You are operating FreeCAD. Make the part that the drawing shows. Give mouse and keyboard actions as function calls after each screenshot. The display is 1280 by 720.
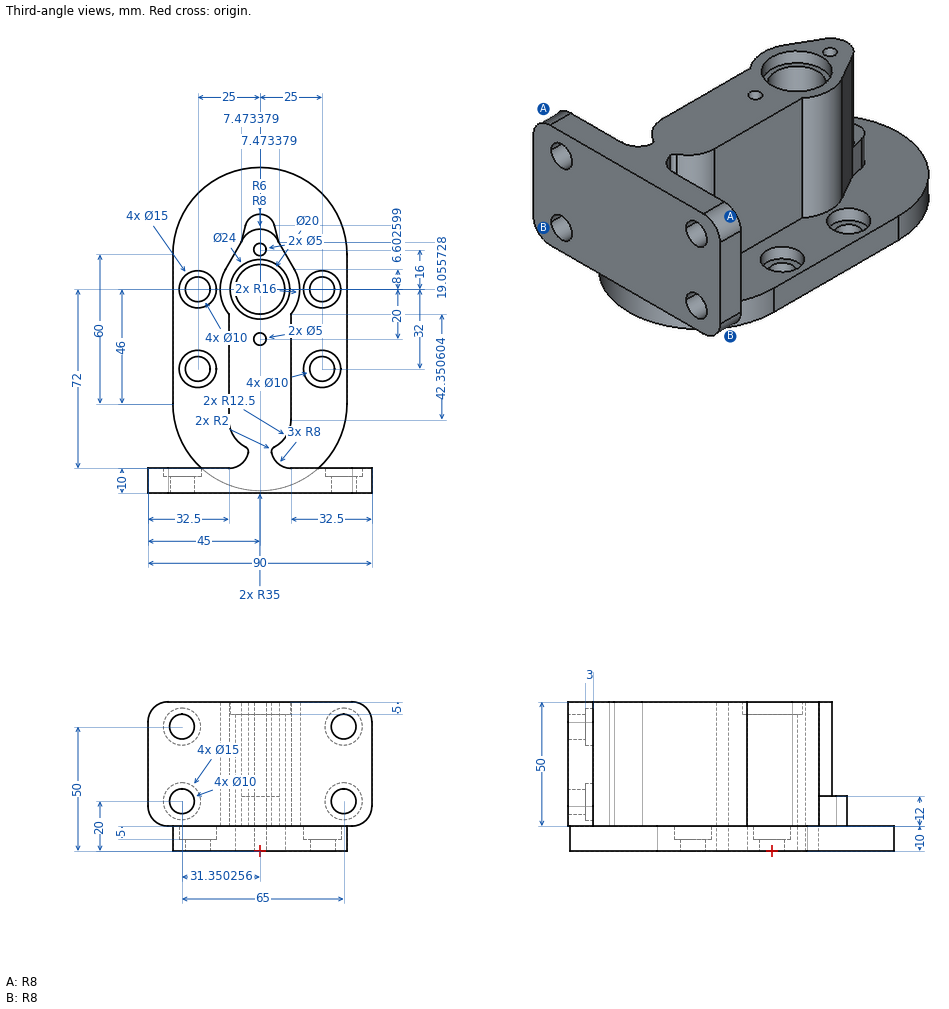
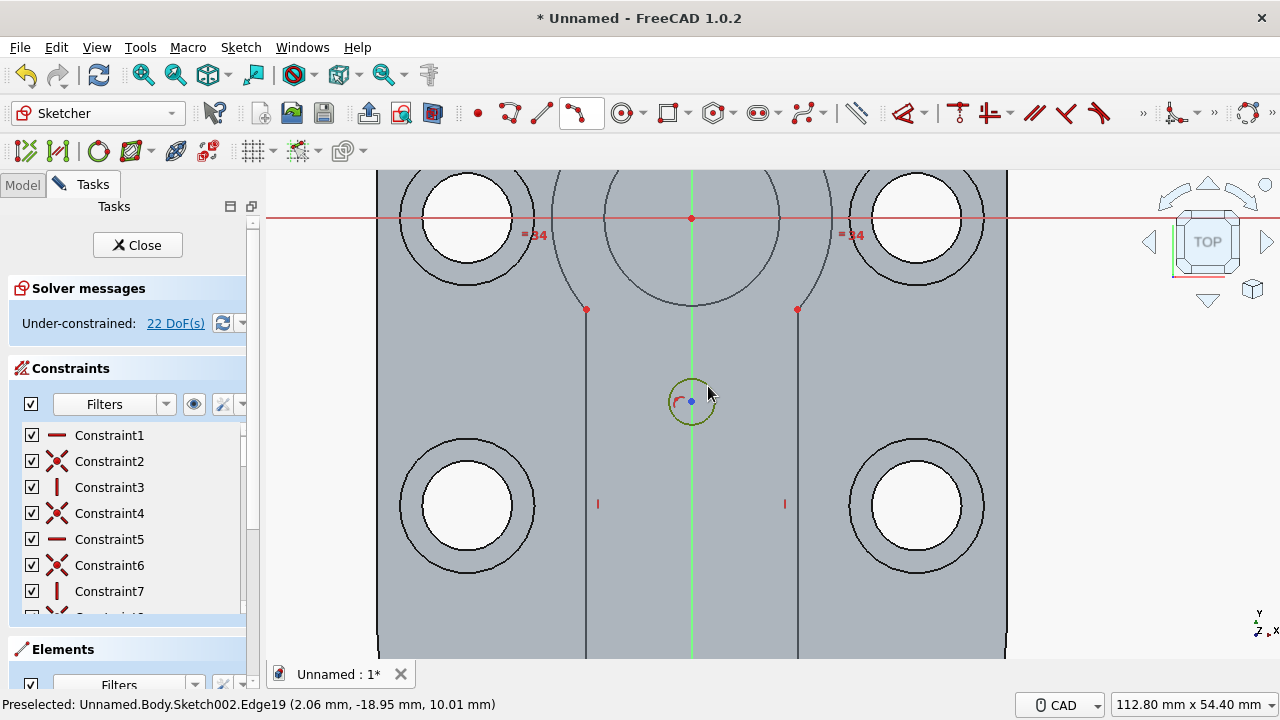
scroll(710, 387, down, 6)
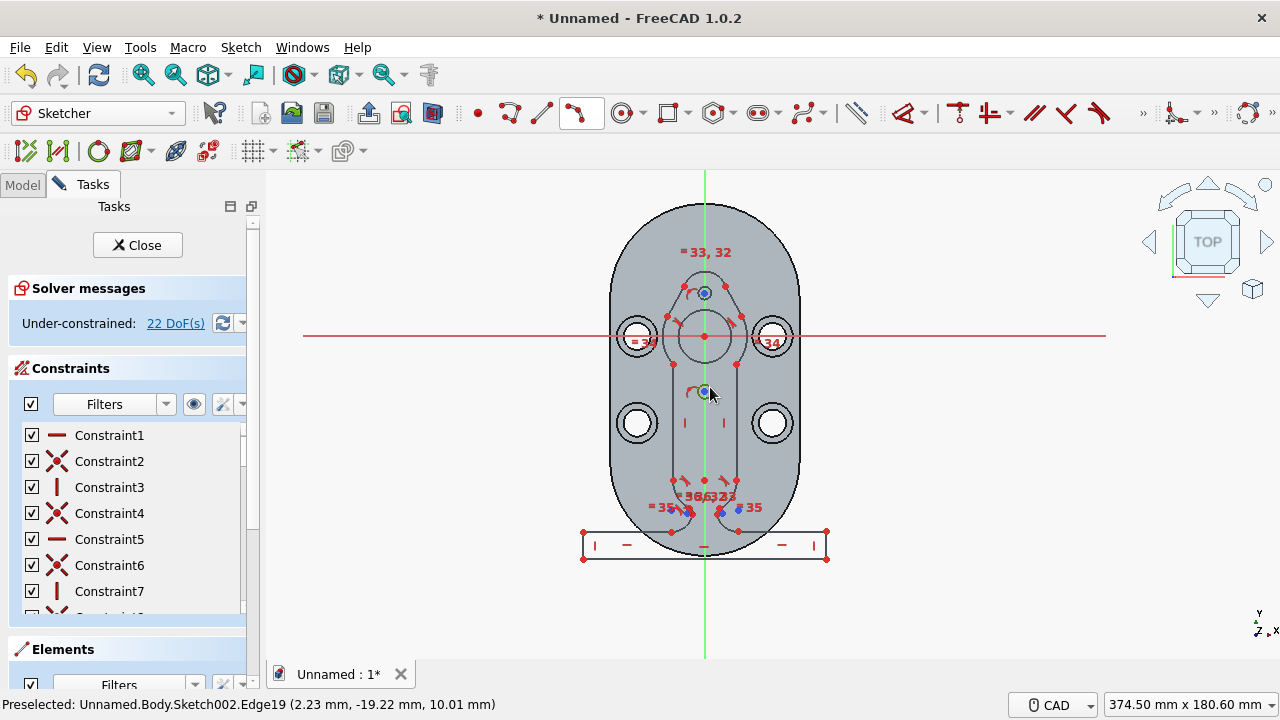
scroll(709, 289, up, 6)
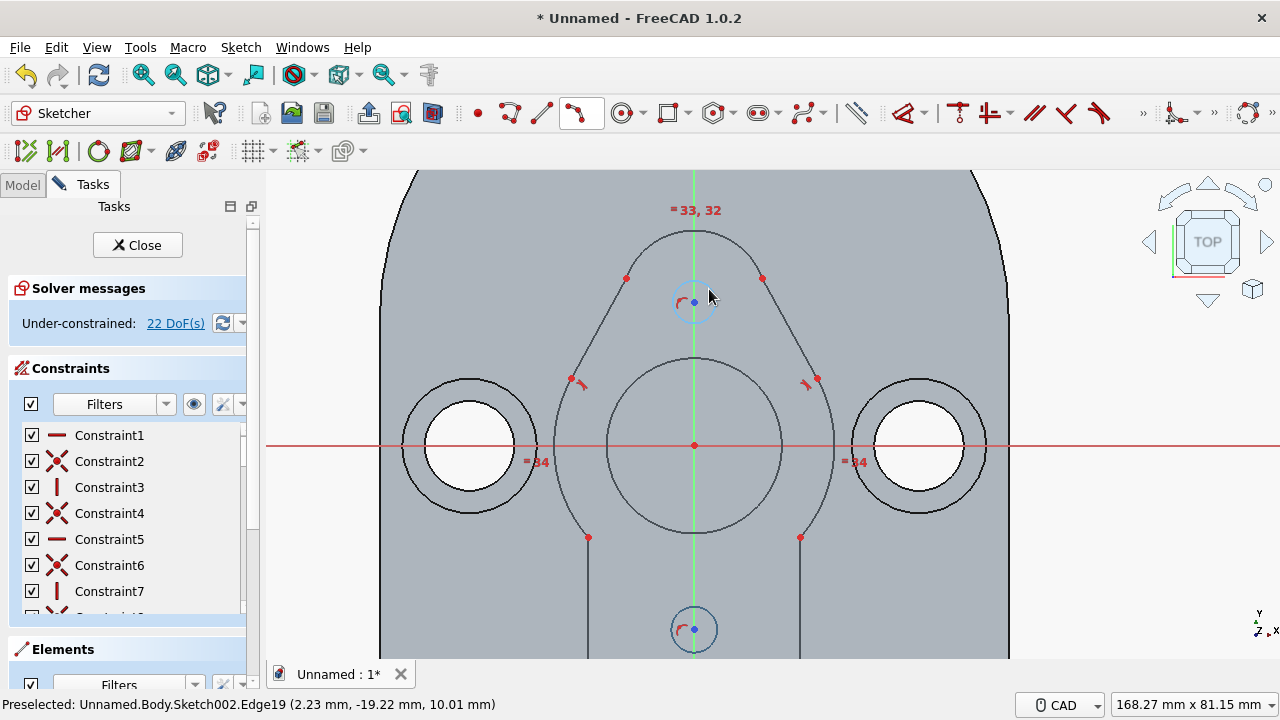
click(709, 287)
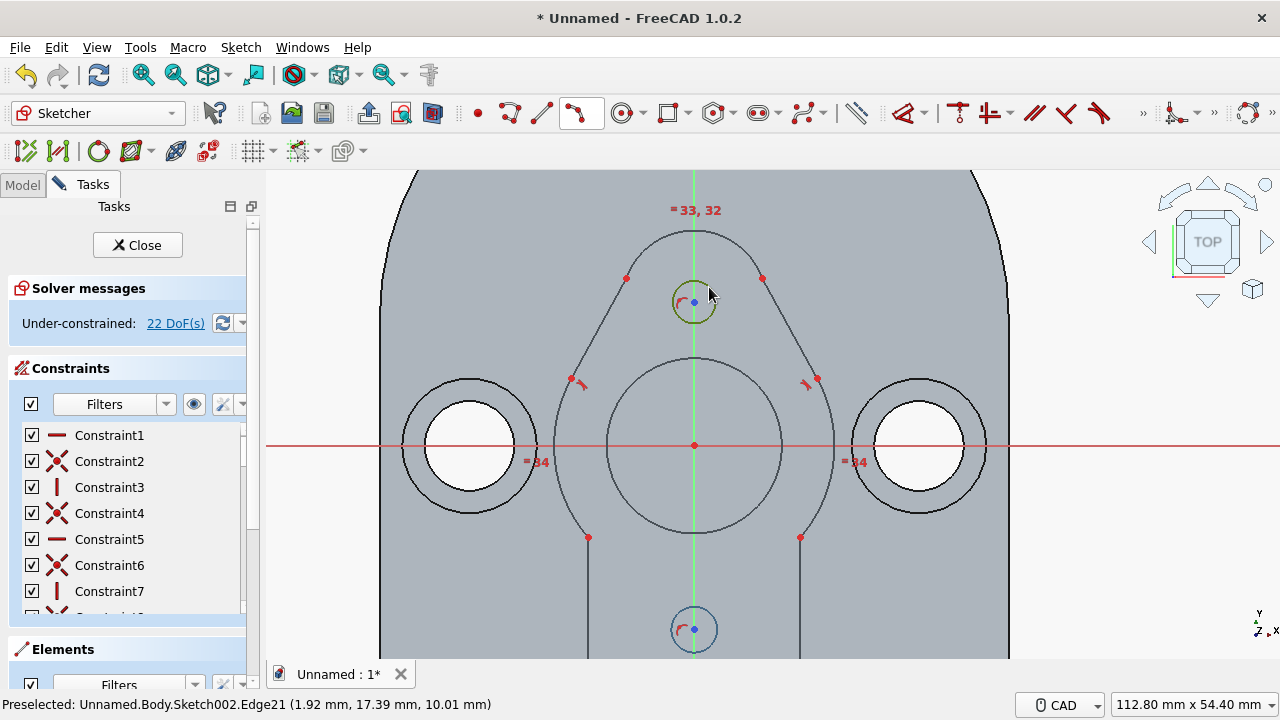
key(e)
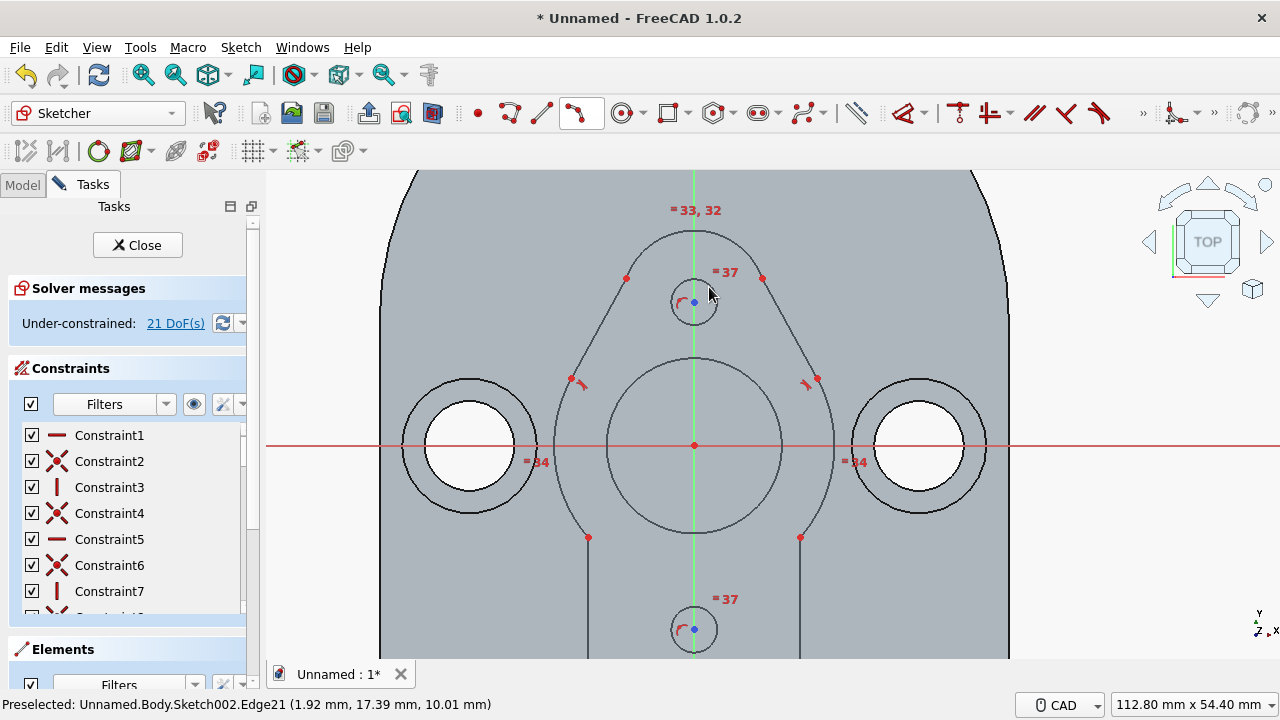
scroll(709, 289, down, 6)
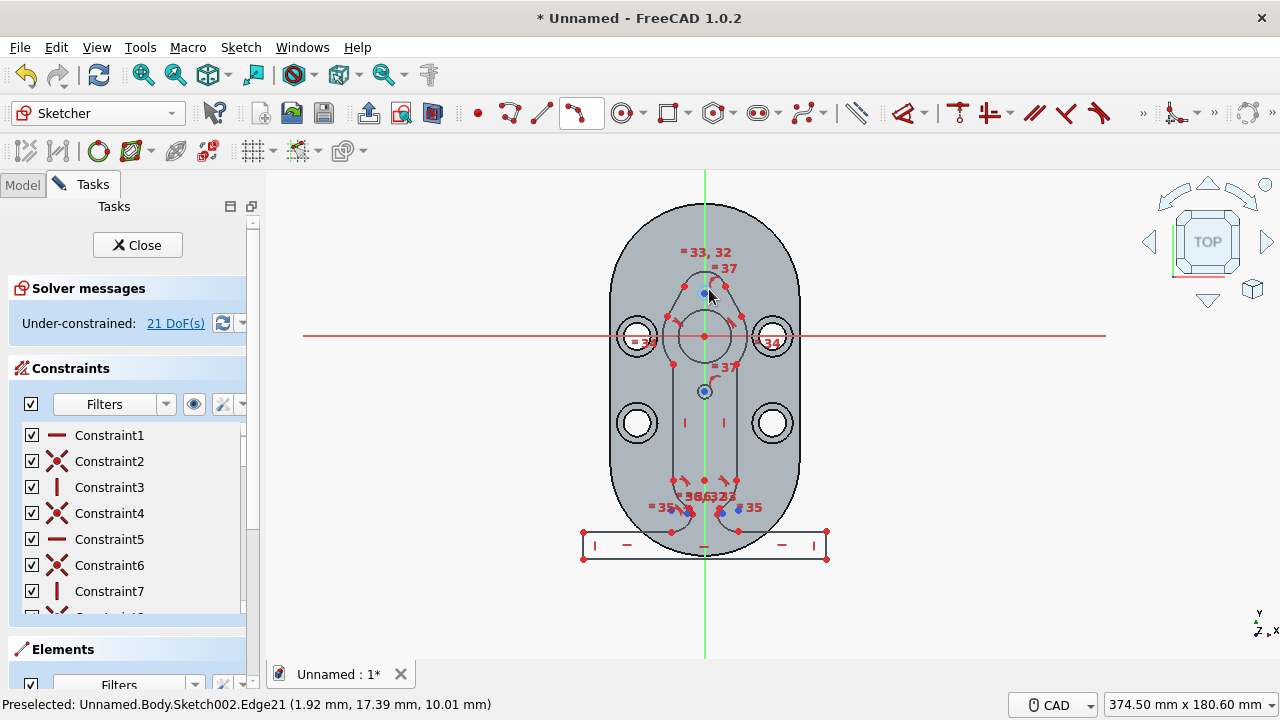
click(705, 481)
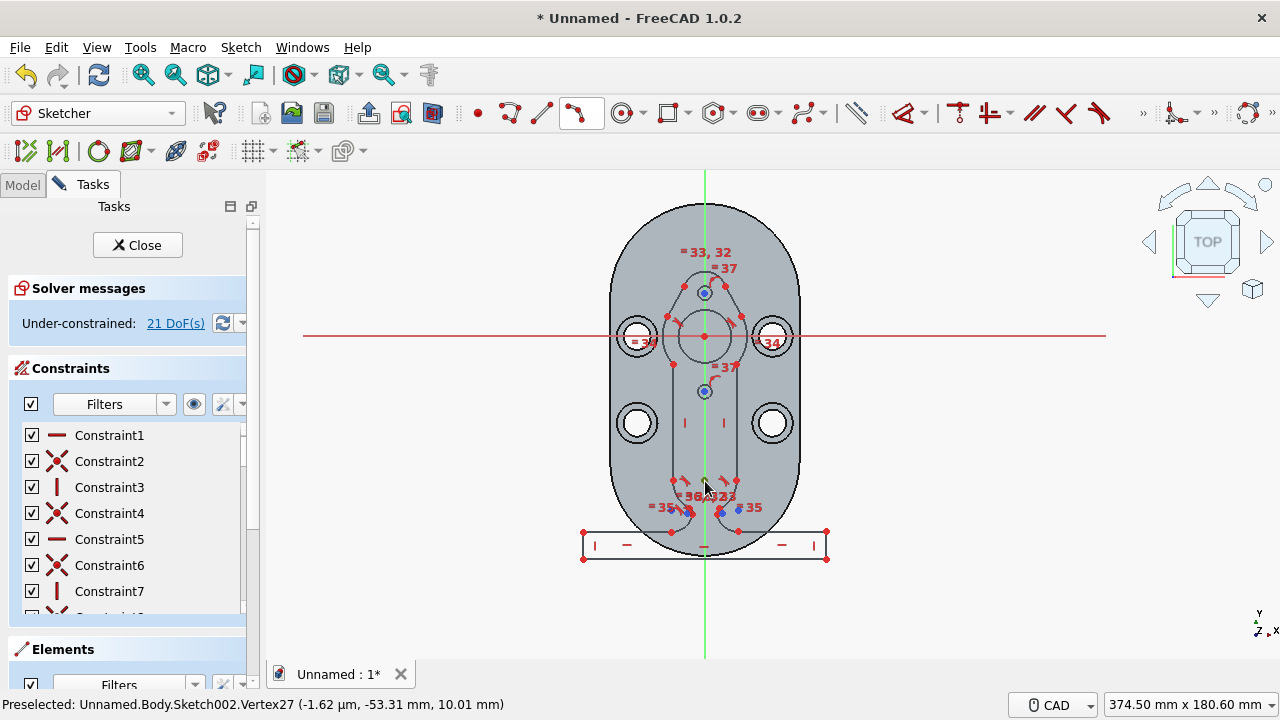
click(705, 600)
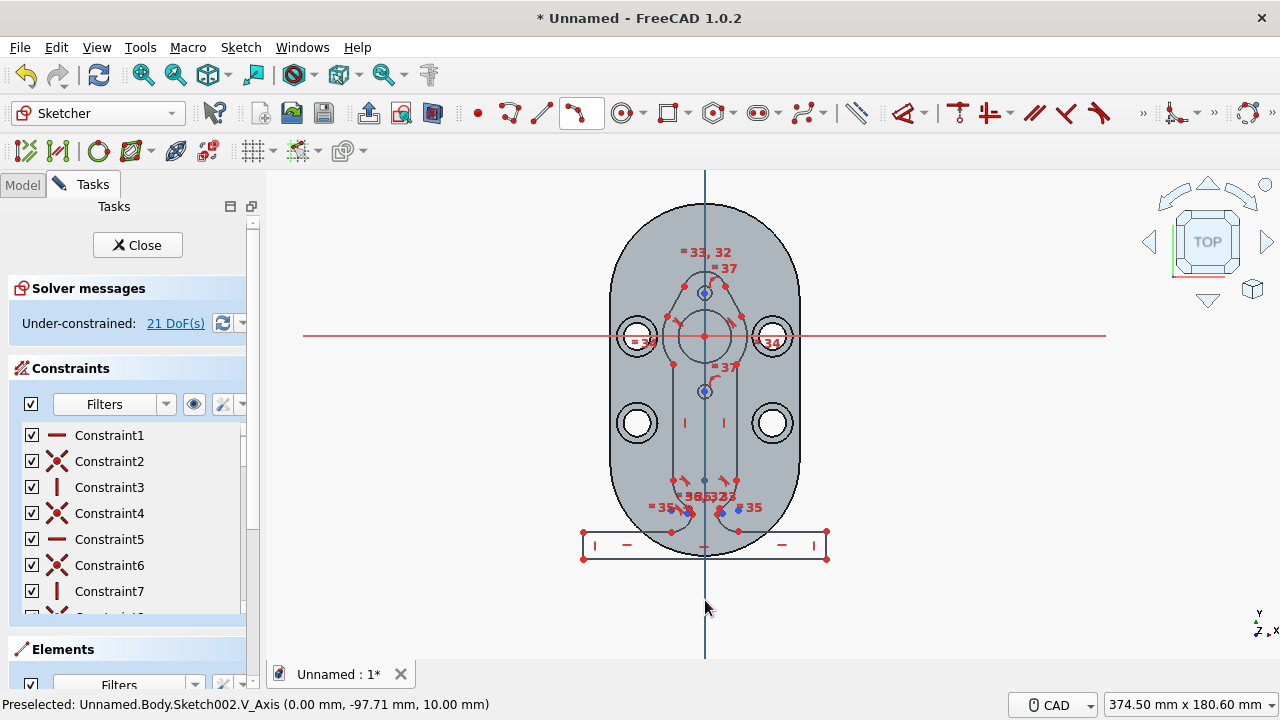
click(958, 114)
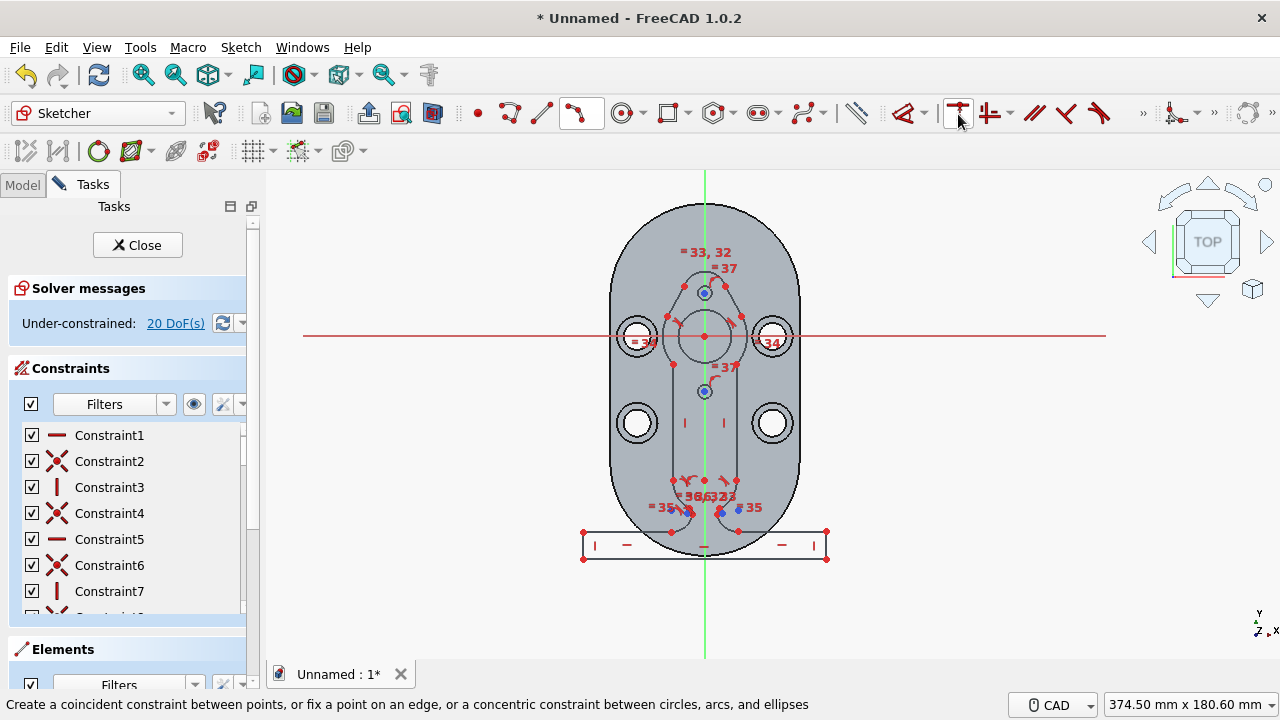
scroll(705, 293, up, 14)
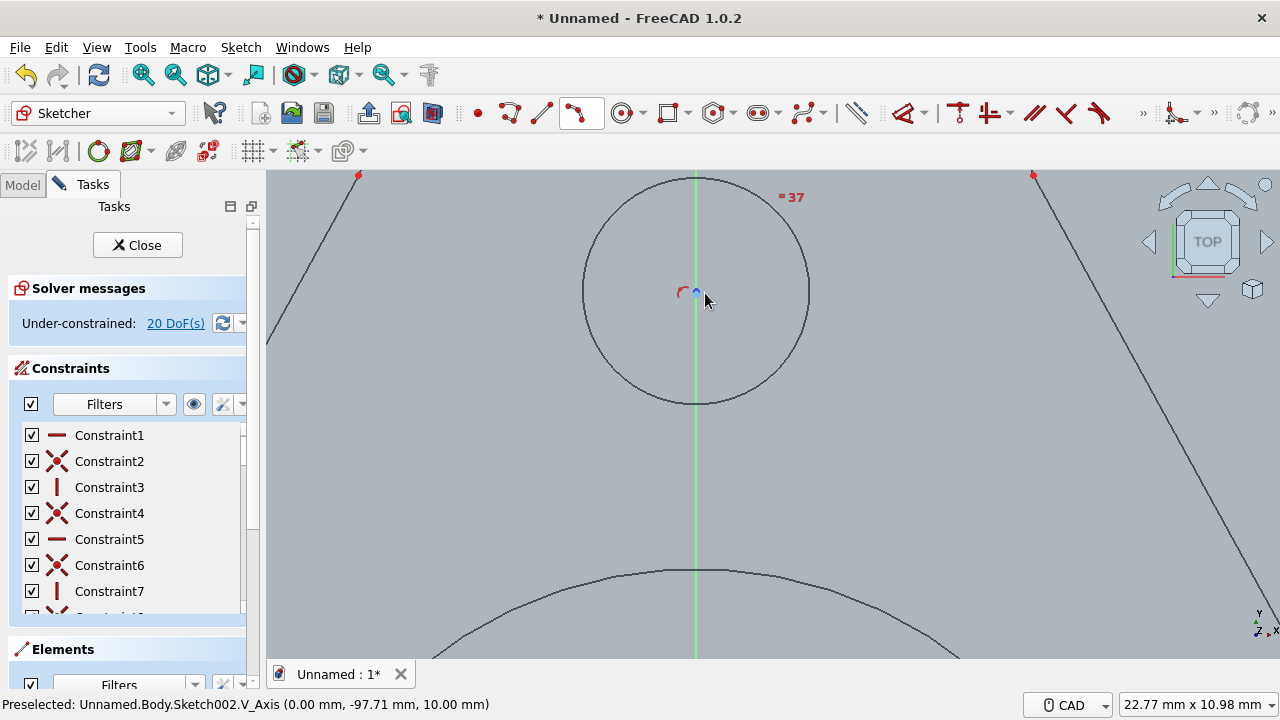
click(696, 294)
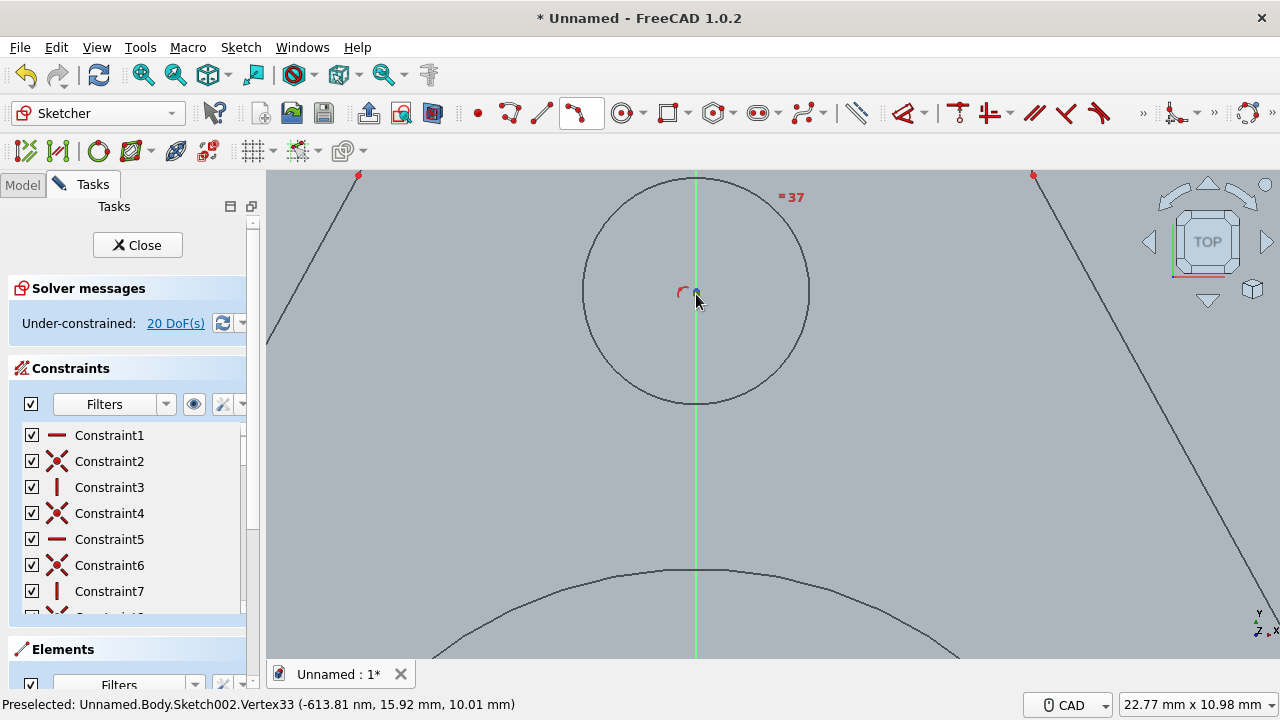
click(696, 600)